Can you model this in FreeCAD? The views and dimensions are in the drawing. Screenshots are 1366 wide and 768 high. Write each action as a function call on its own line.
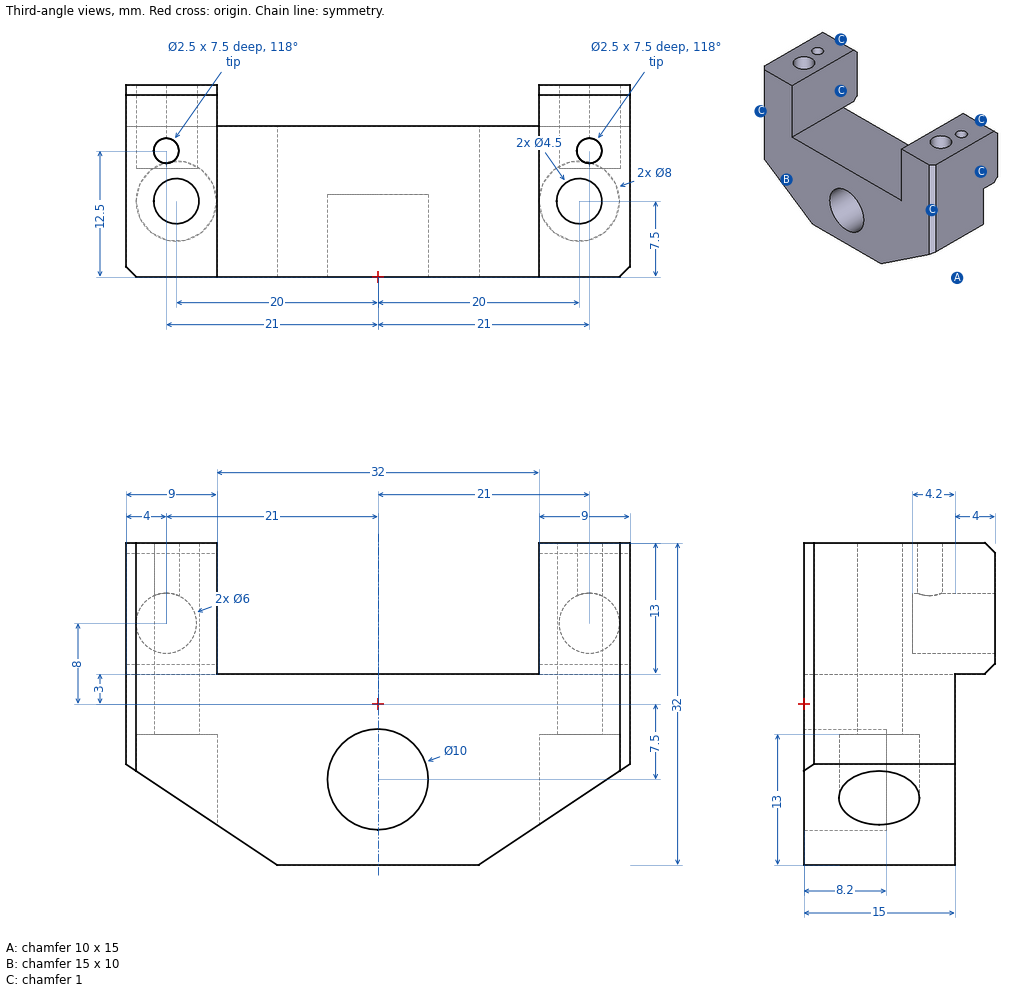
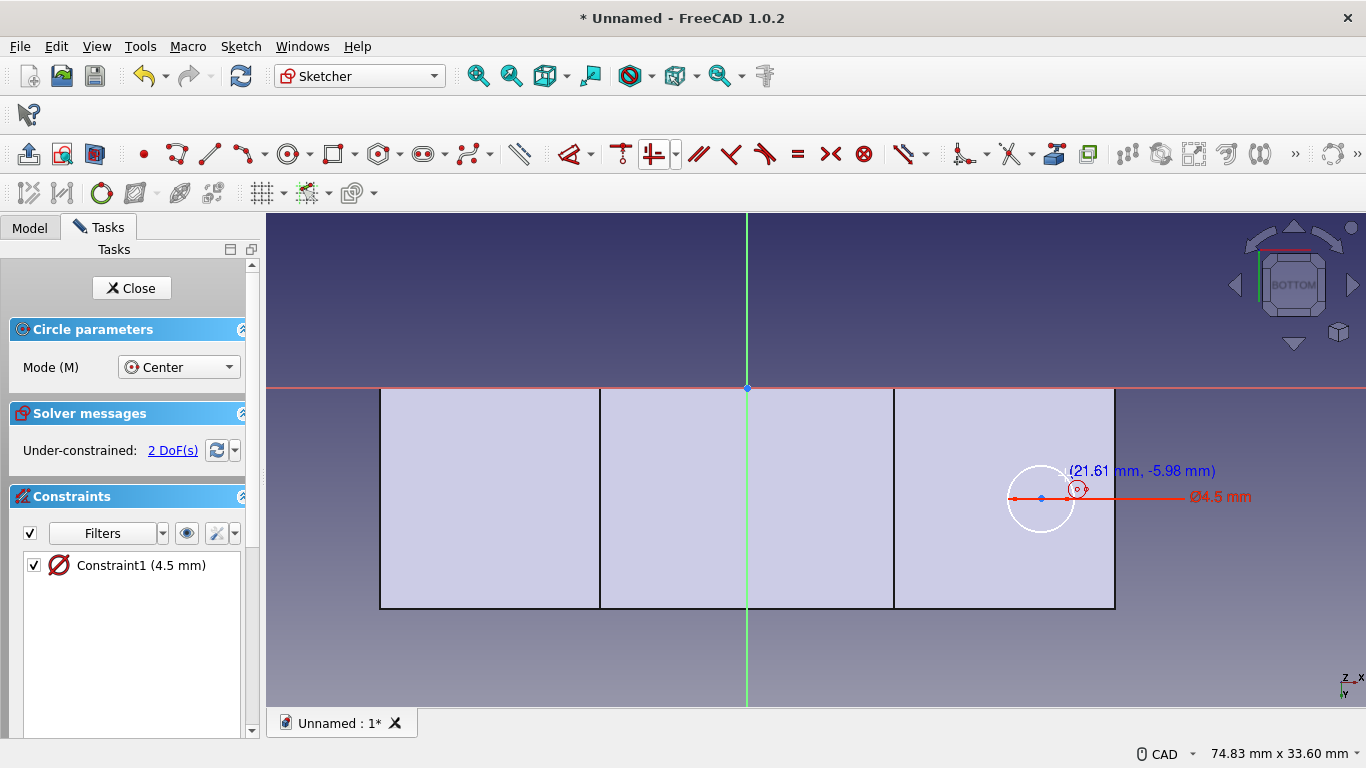
click(453, 498)
move(477, 475)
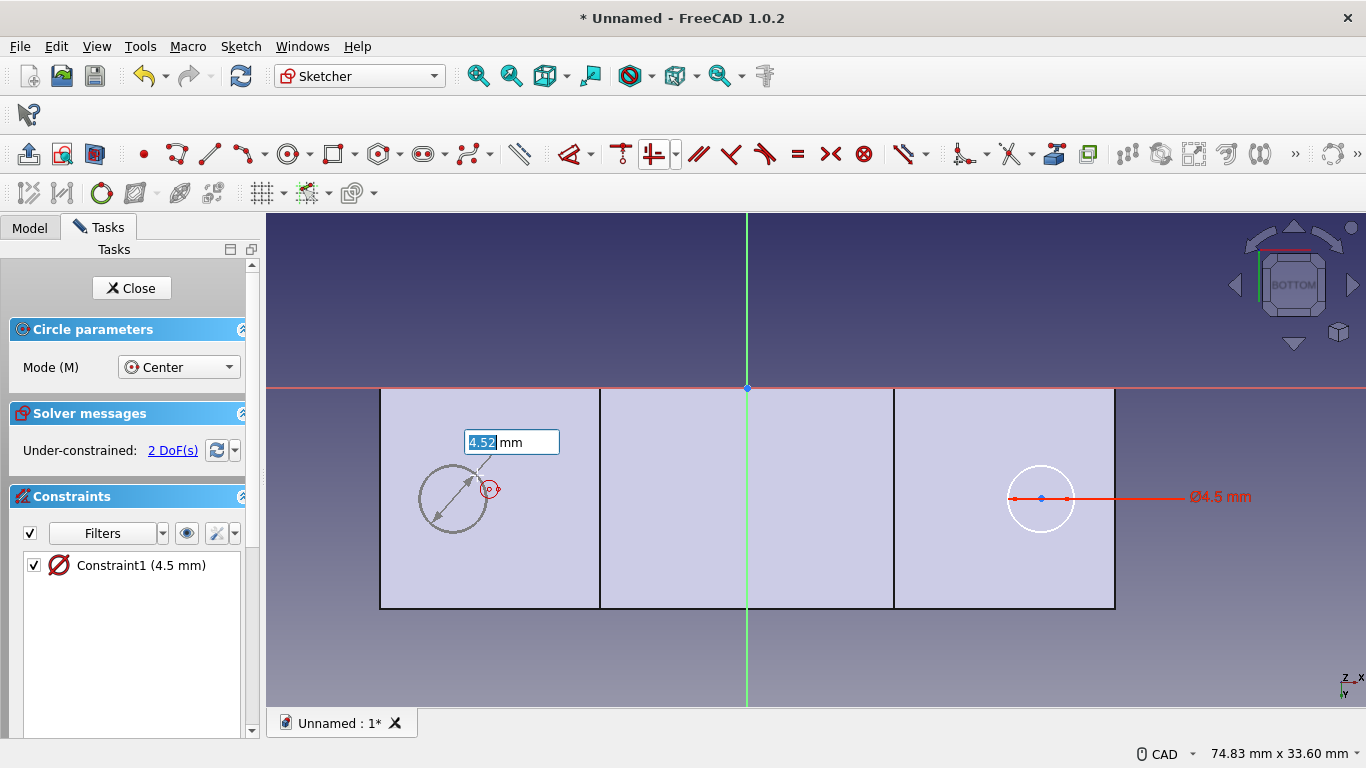
text(4.5)
key(Return)
key(Escape)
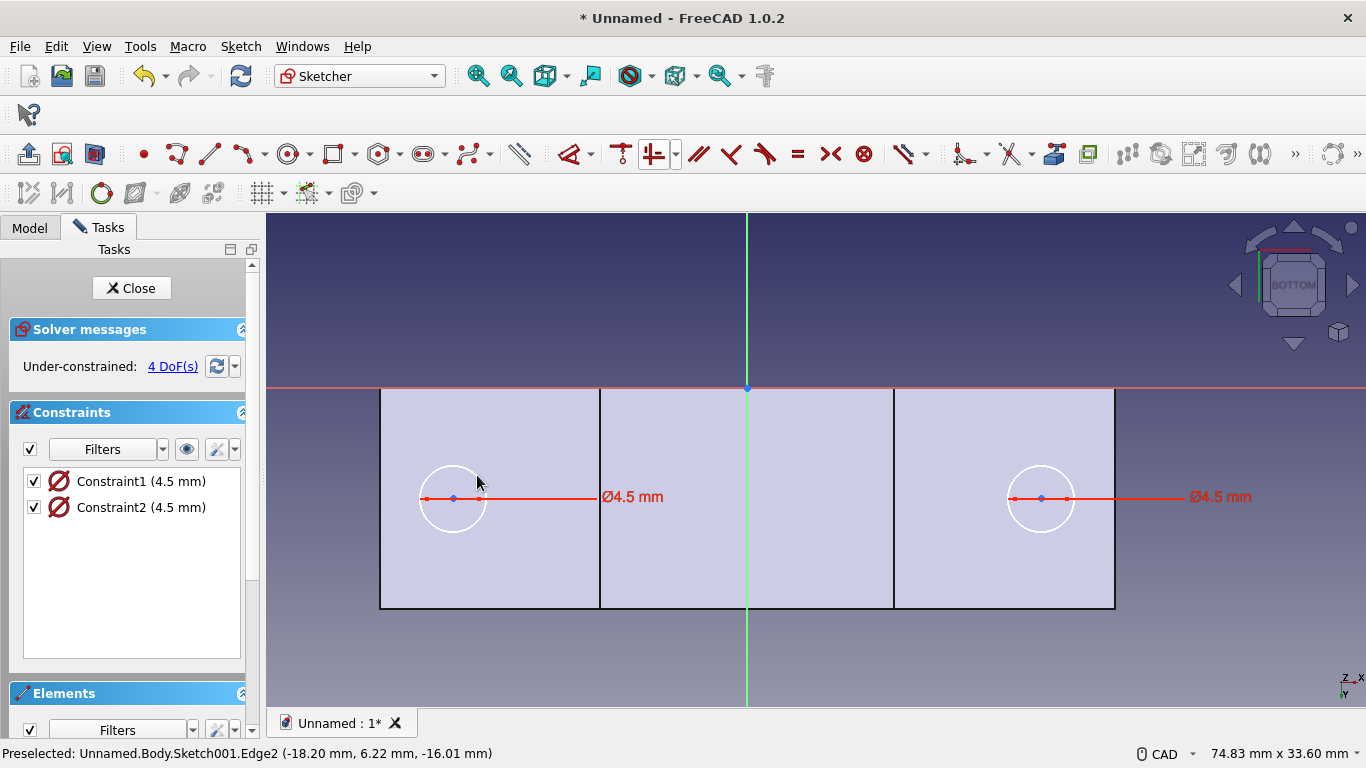
click(1041, 499)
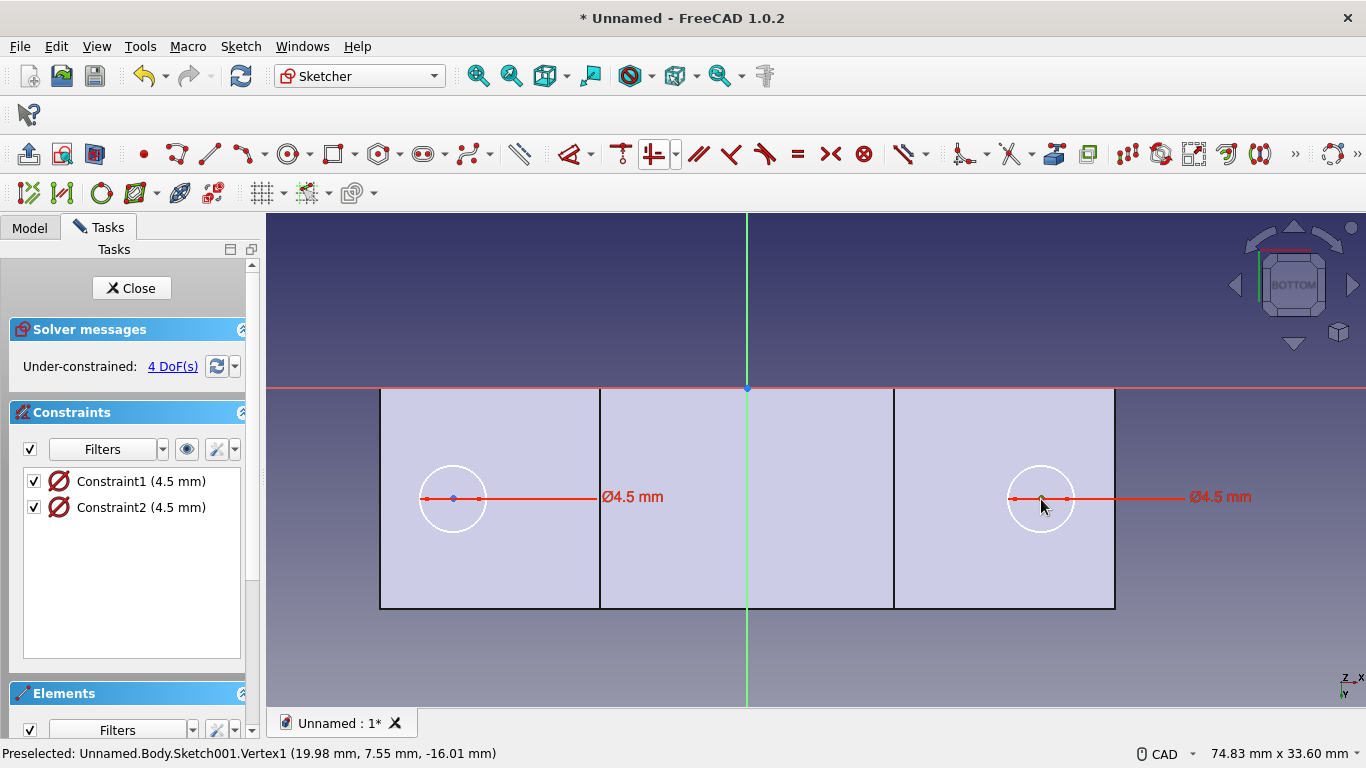
click(453, 499)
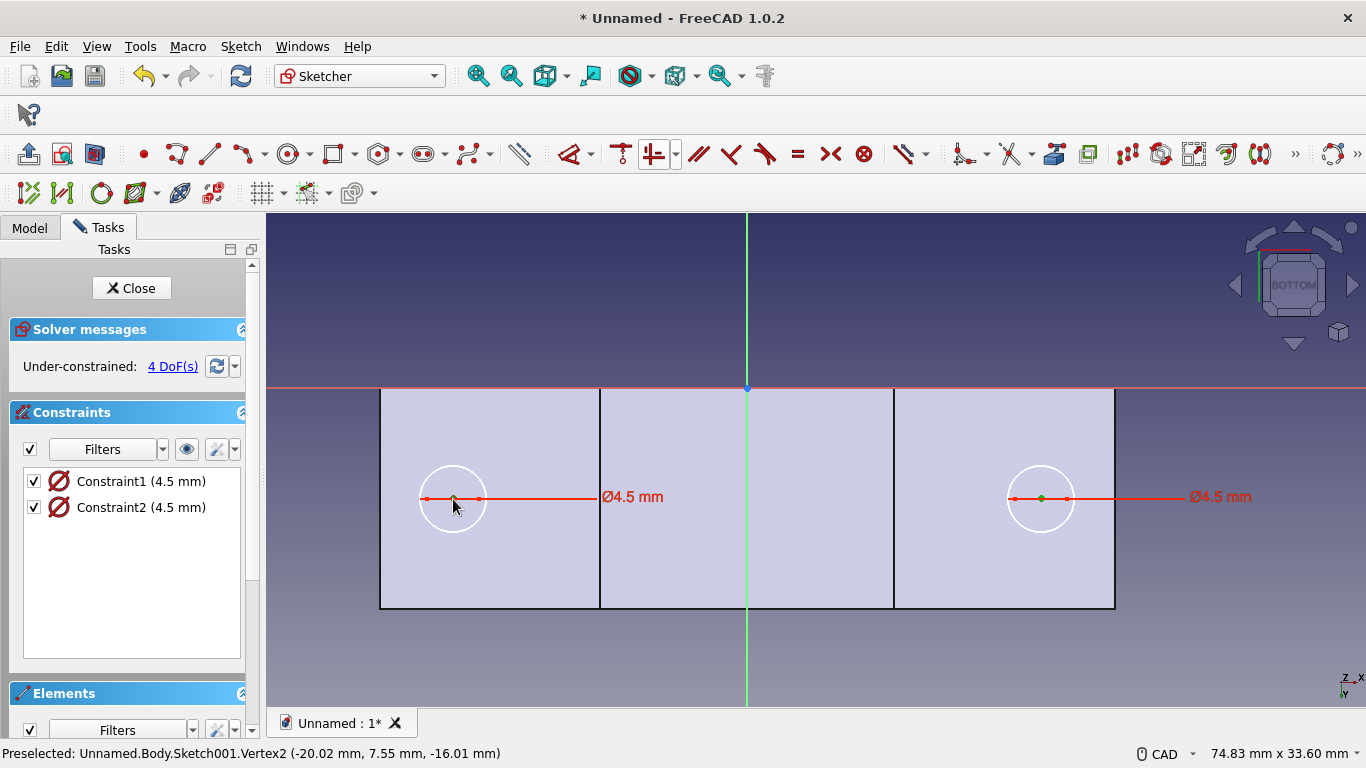
click(676, 154)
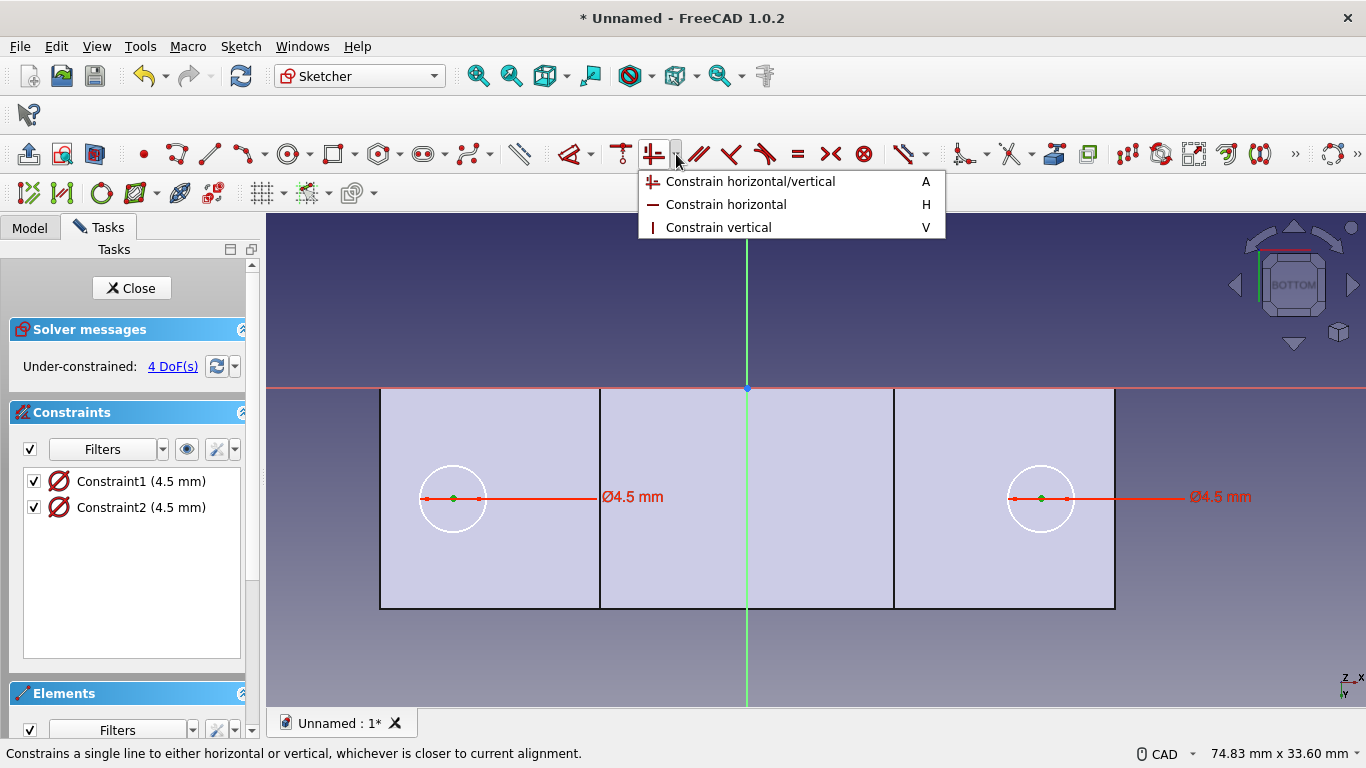
click(792, 204)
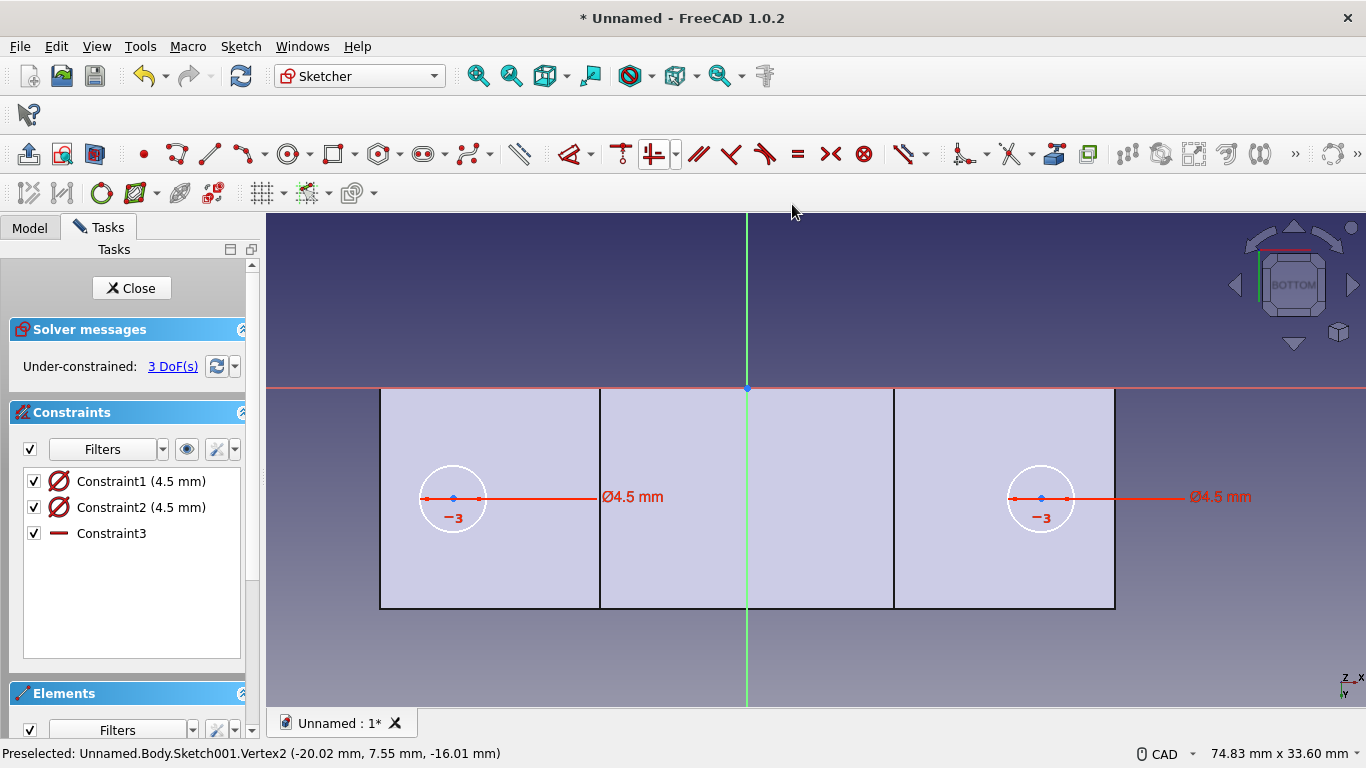
click(568, 154)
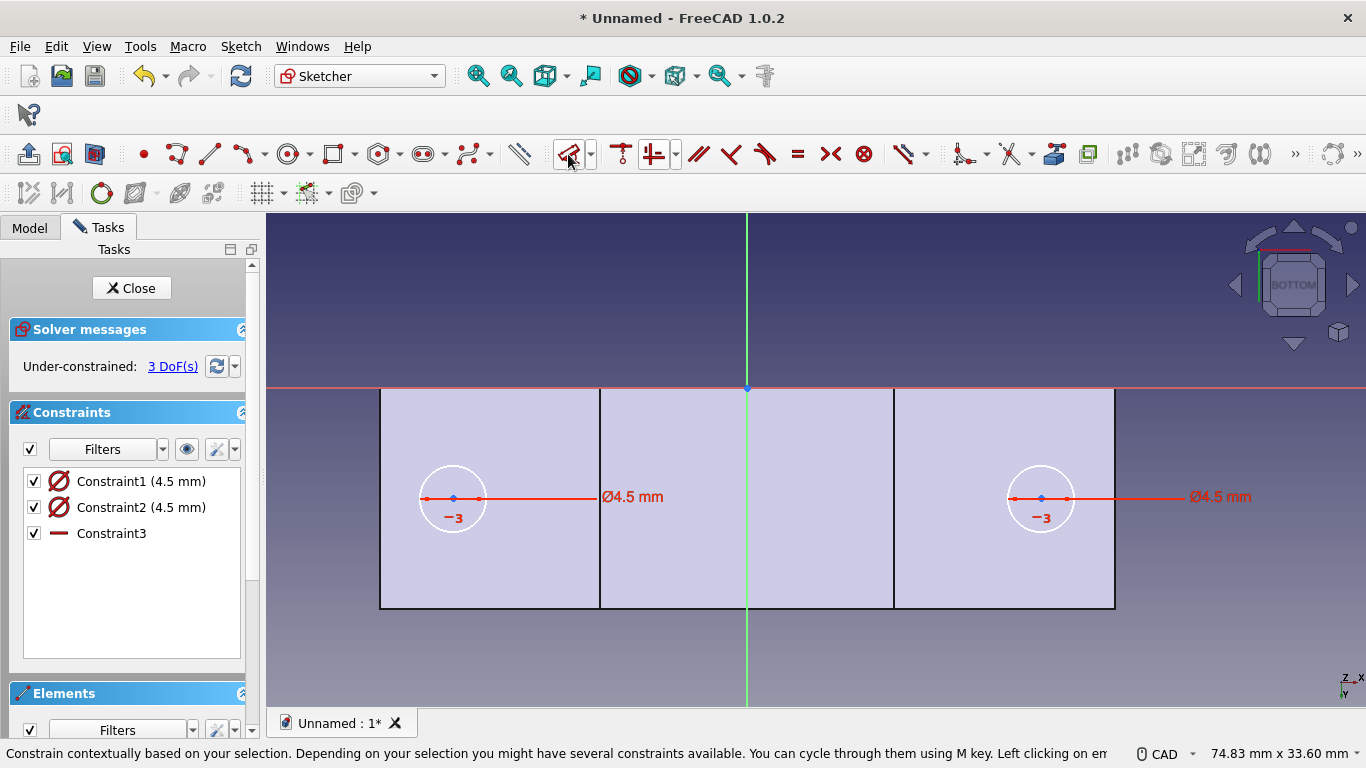
click(1041, 499)
click(894, 354)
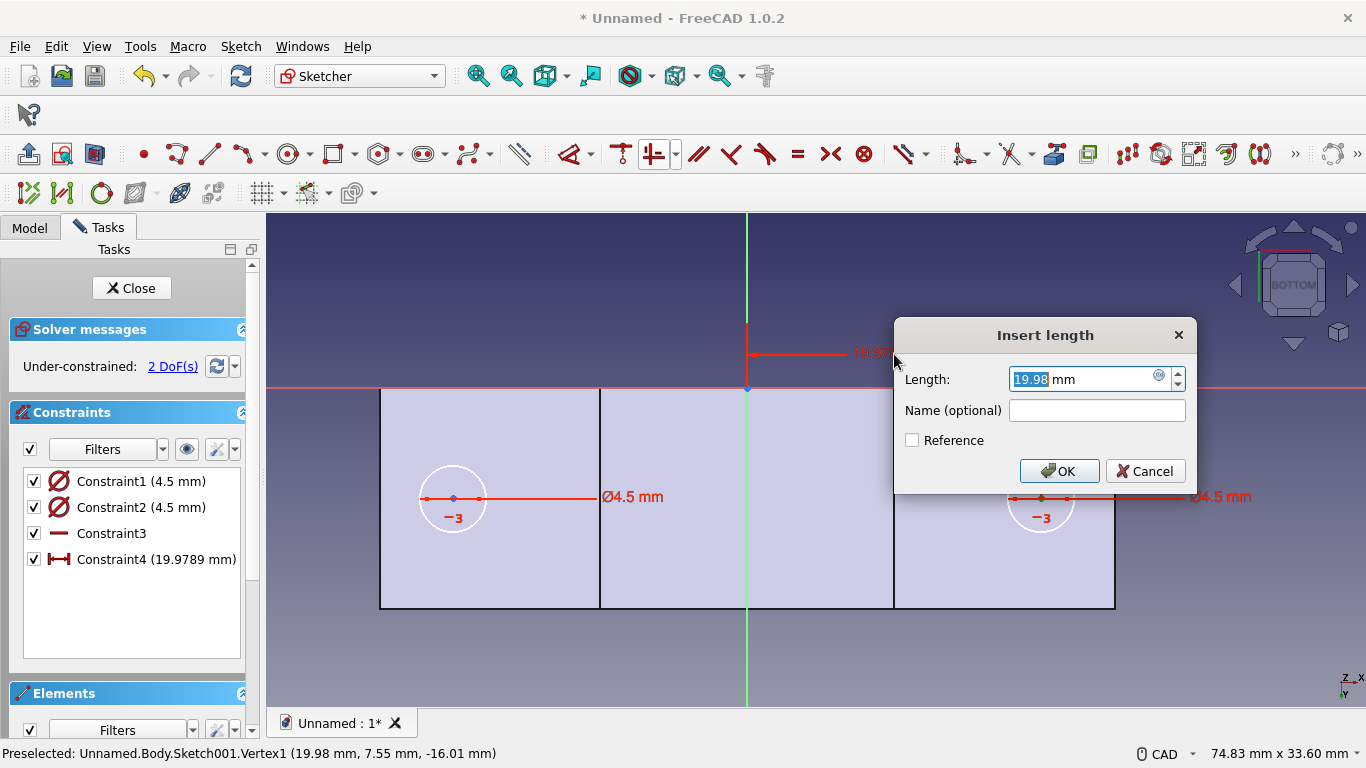
text(20)
key(Return)